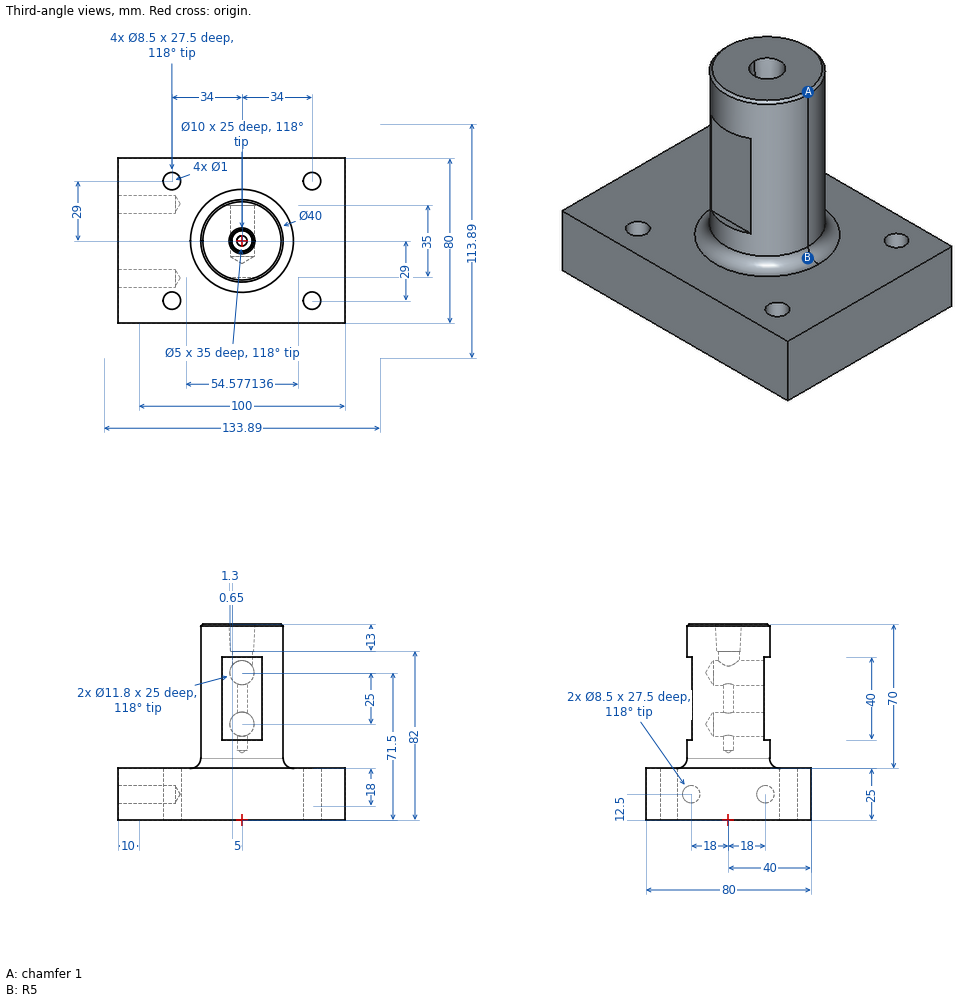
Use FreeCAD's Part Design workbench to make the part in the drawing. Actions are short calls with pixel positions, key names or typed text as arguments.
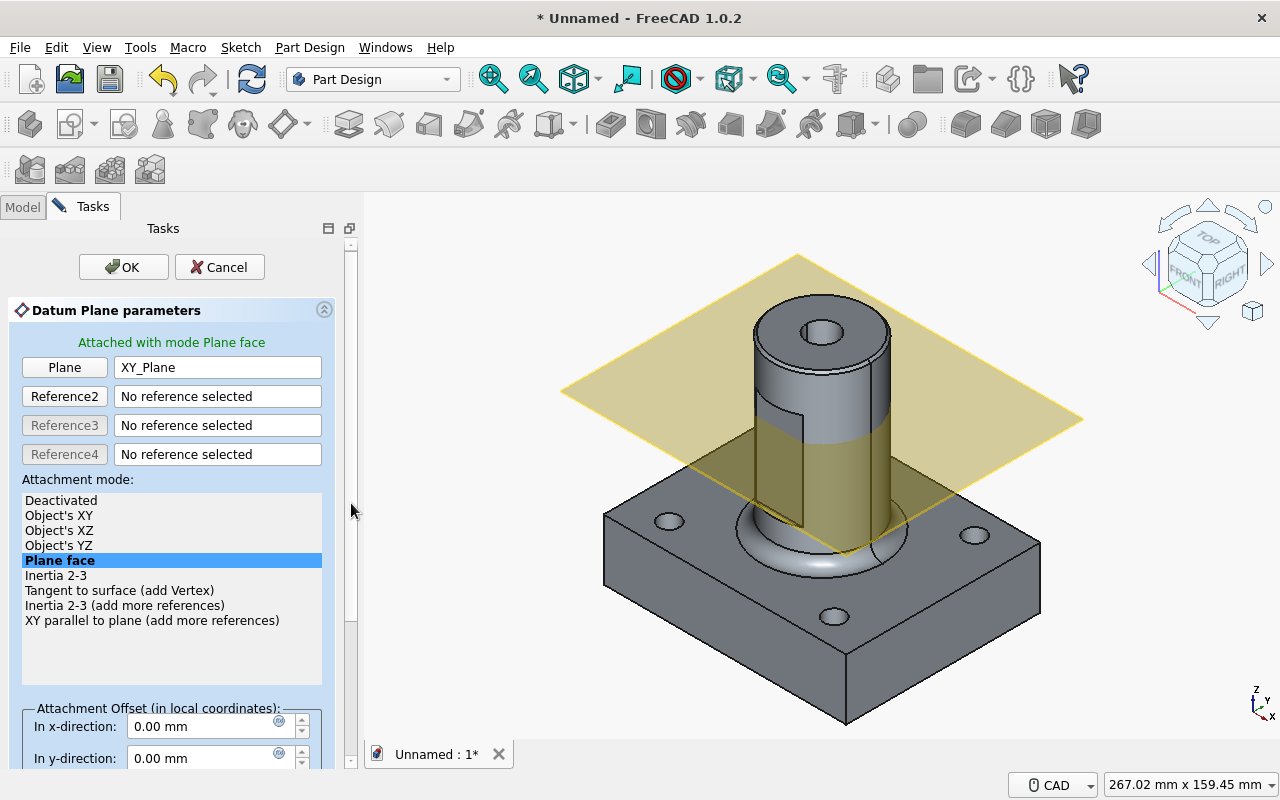
click(124, 267)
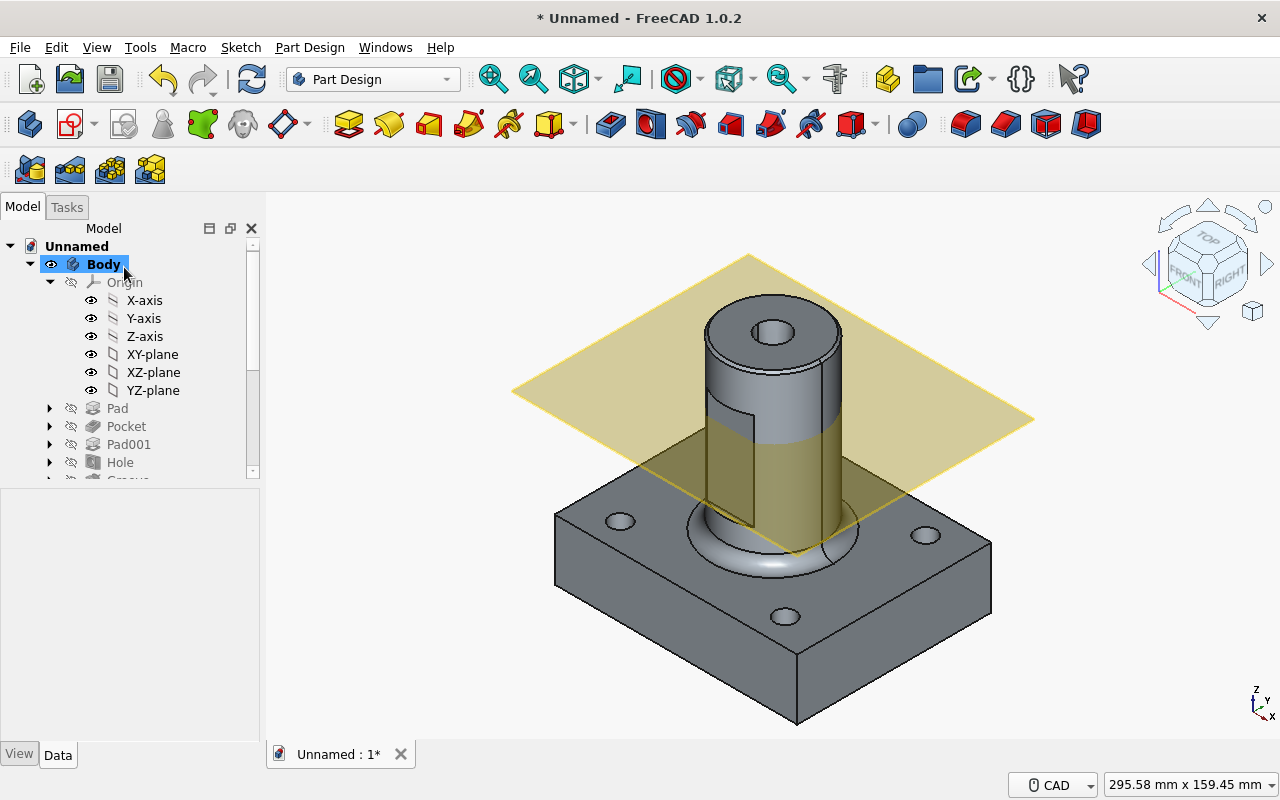
scroll(100, 350, down, 3)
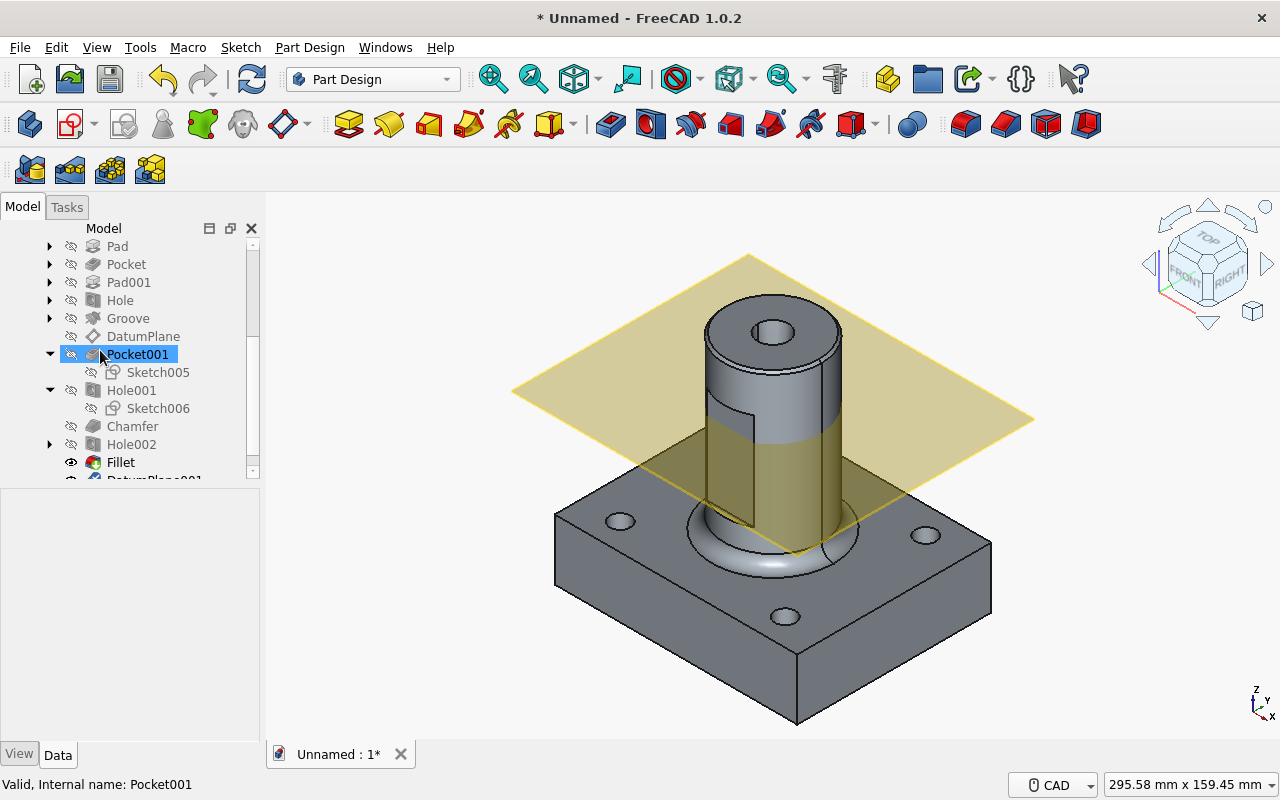
scroll(140, 350, up, 15)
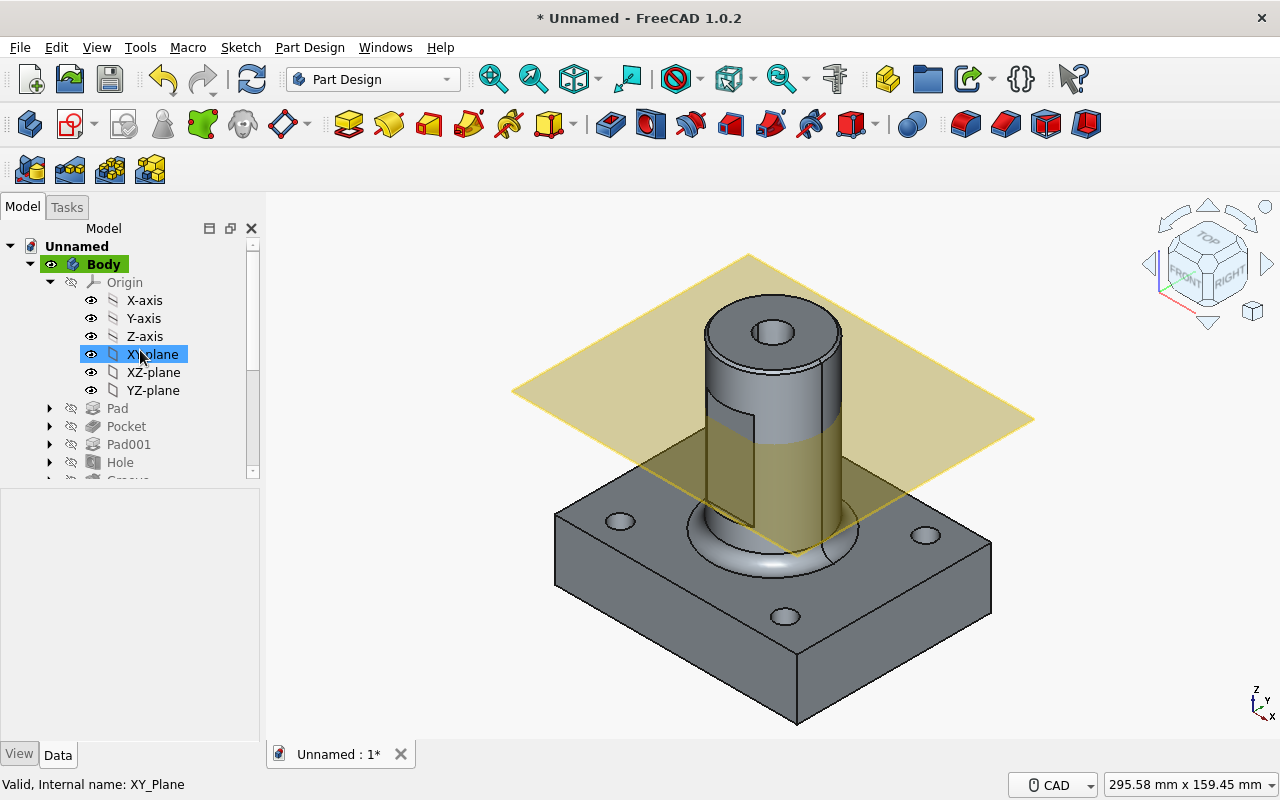
scroll(100, 350, down, 6)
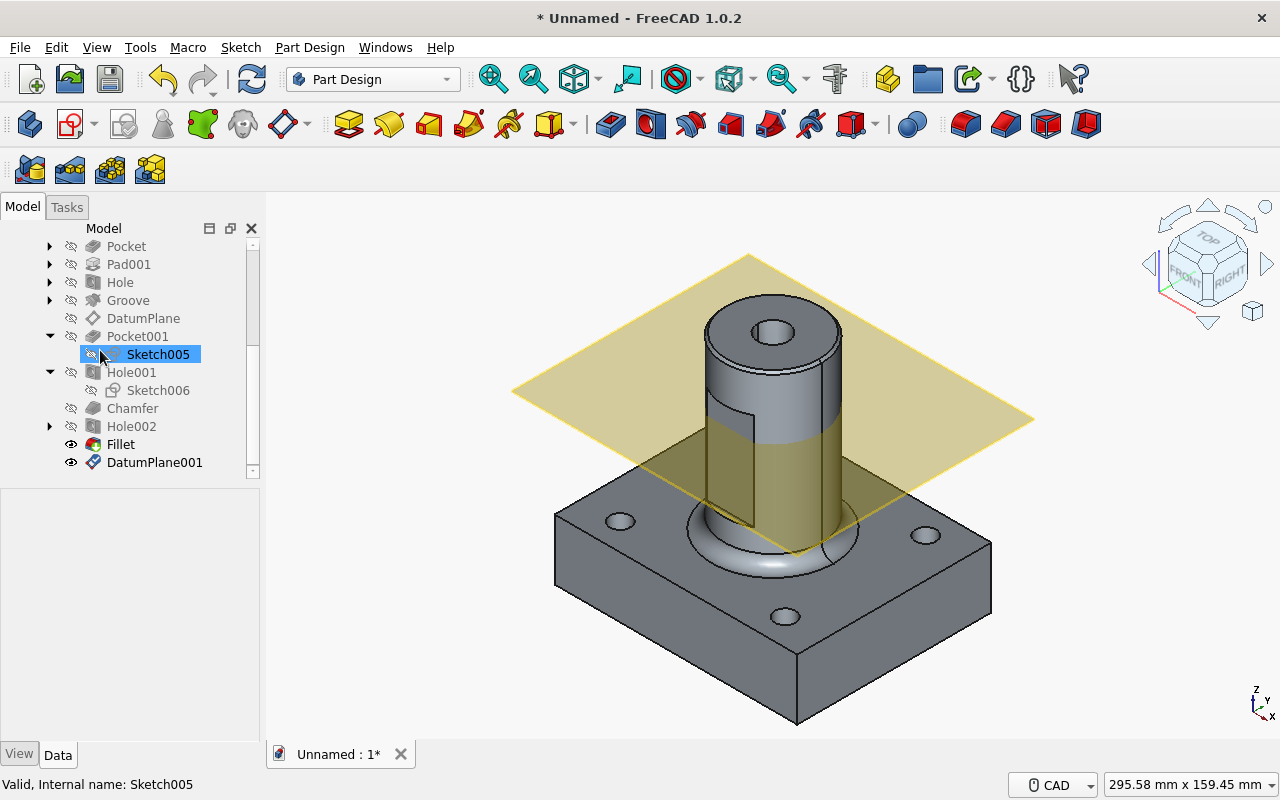
click(116, 462)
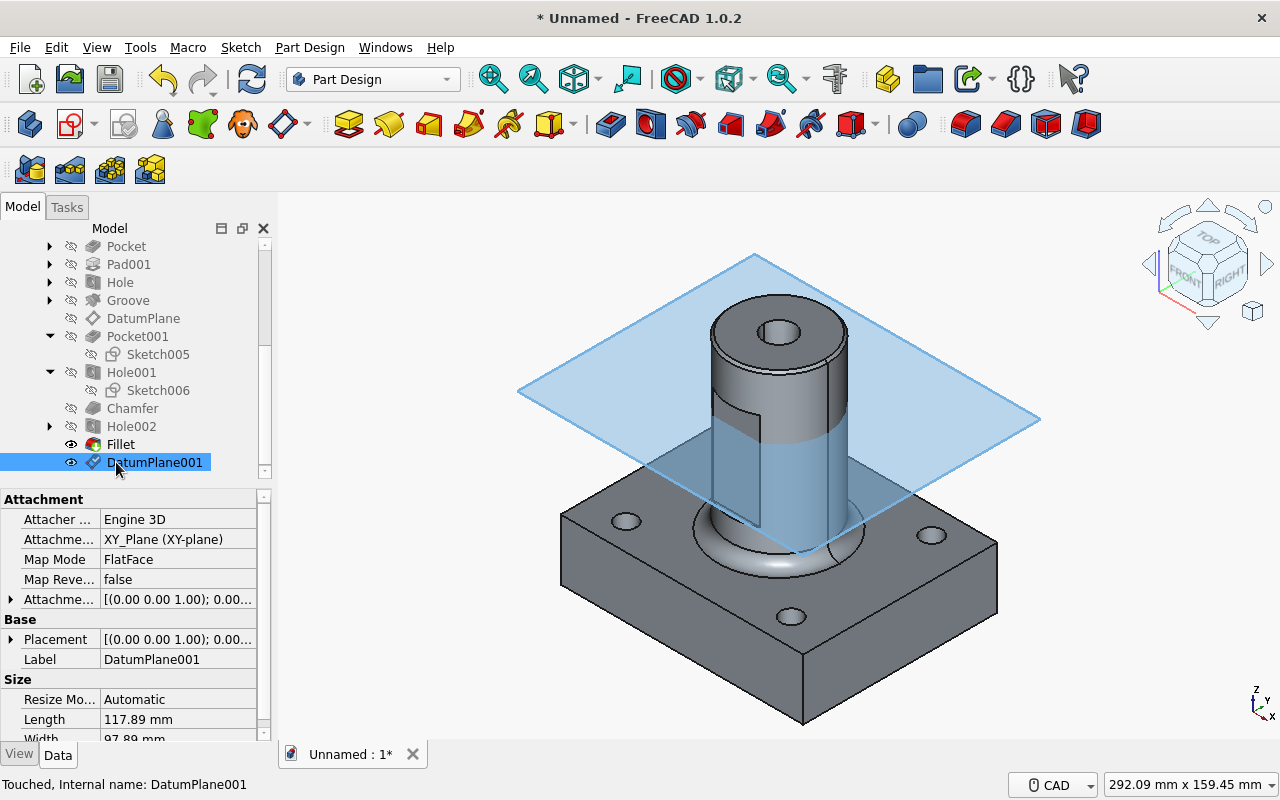
click(70, 124)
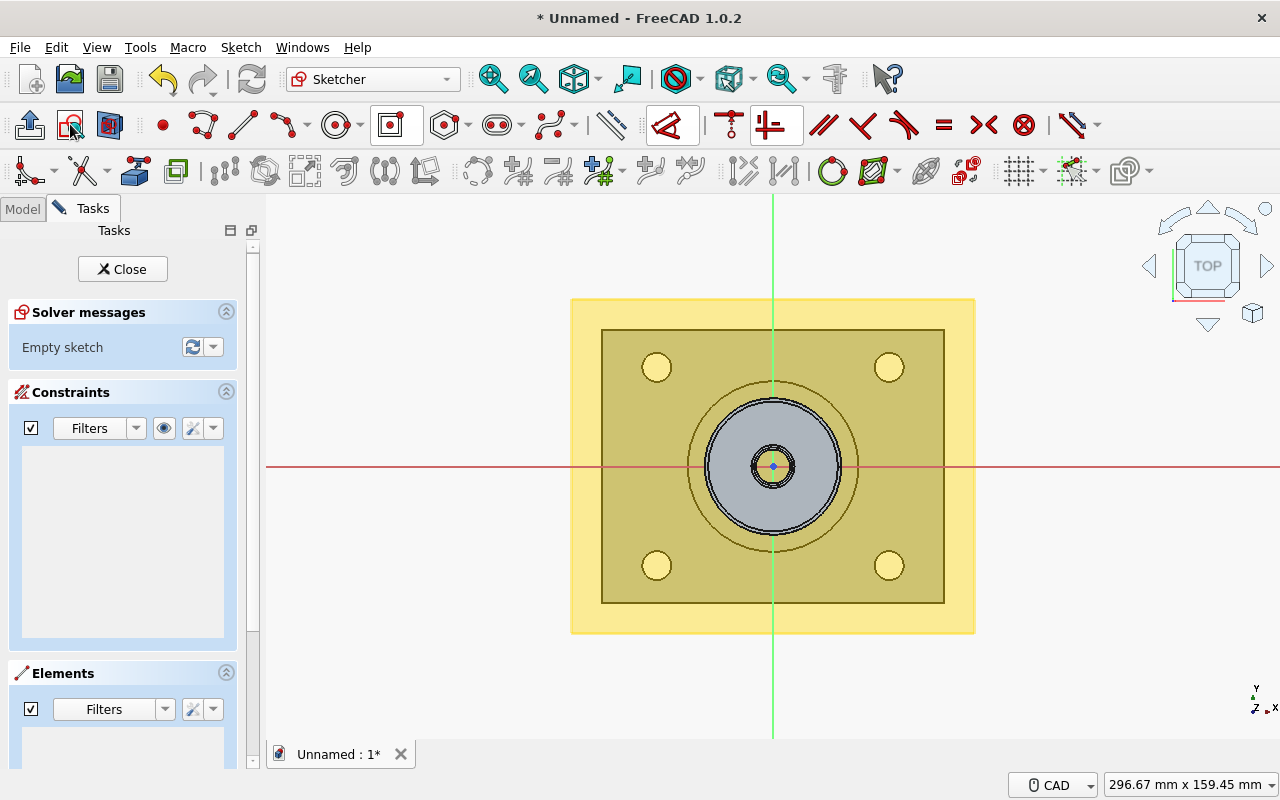
click(110, 126)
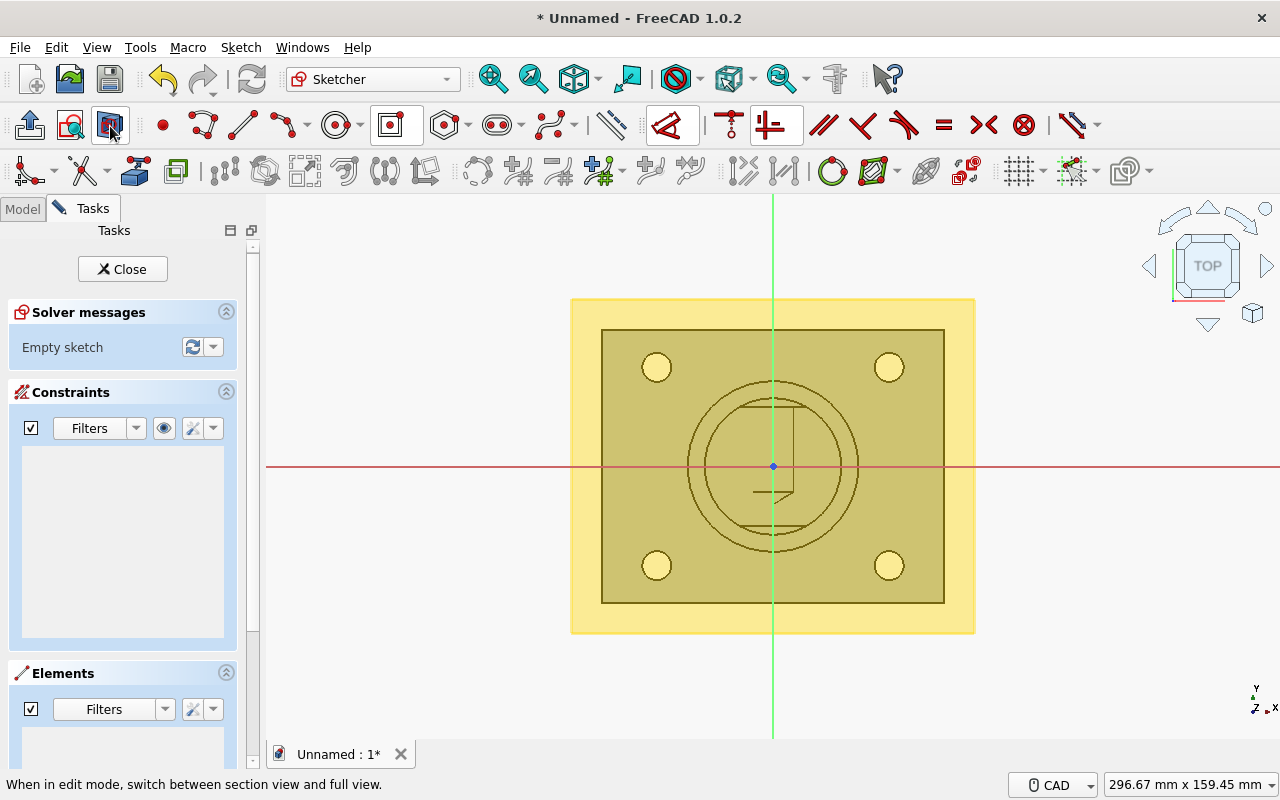
scroll(777, 466, up, 15)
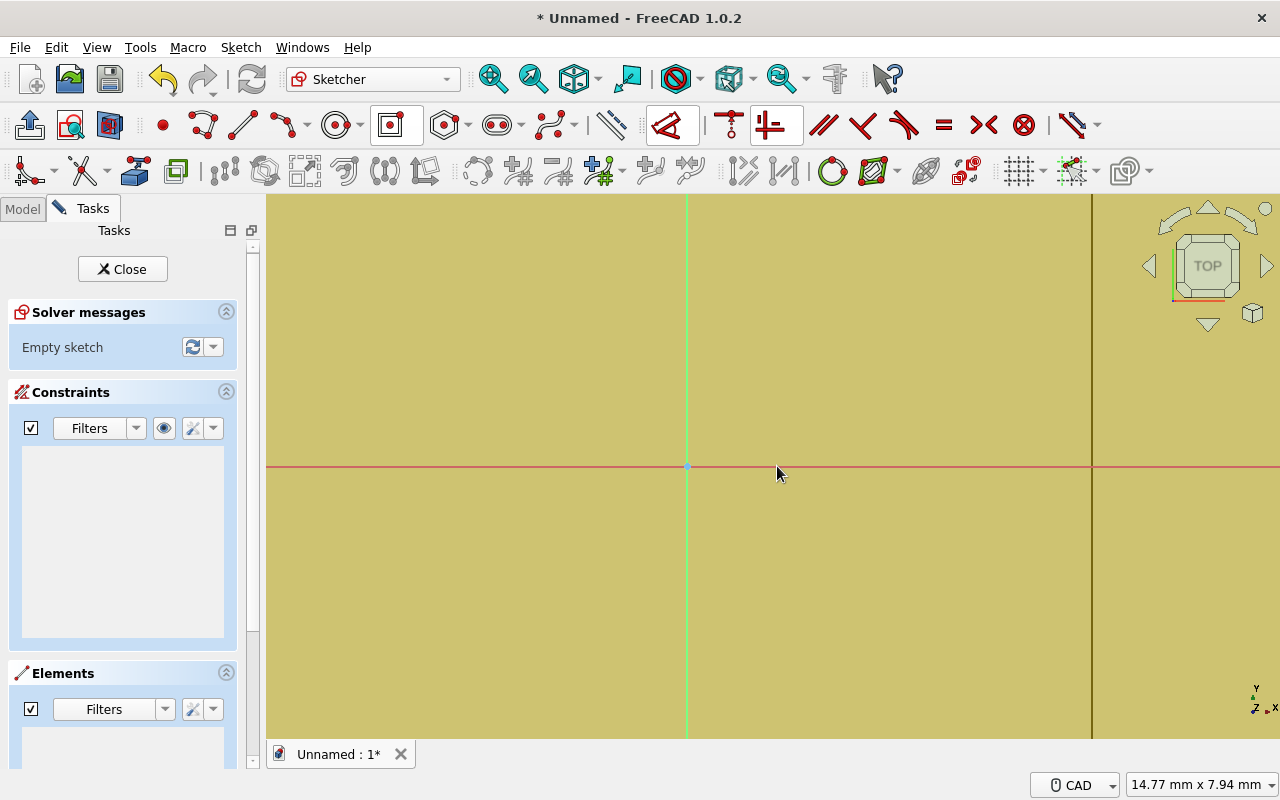
key(g)
key(c)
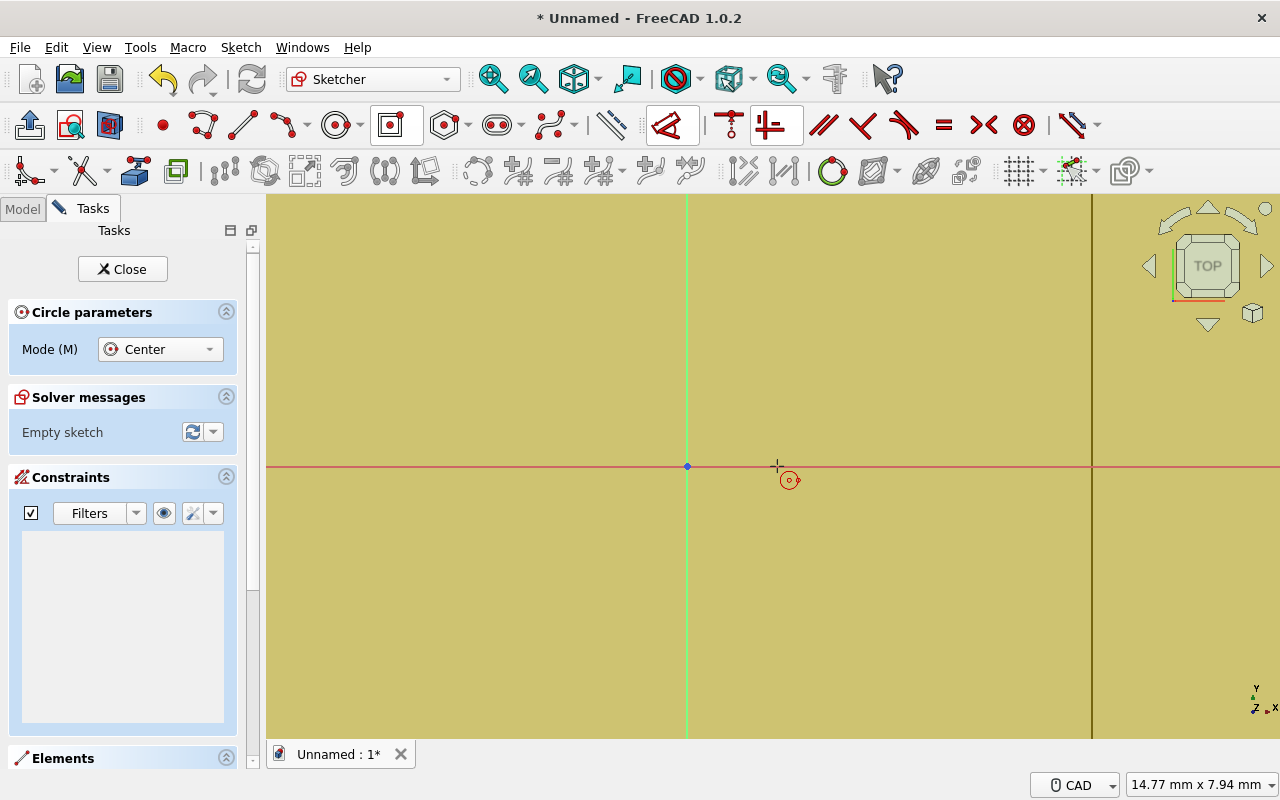
click(687, 466)
click(808, 345)
key(Escape)